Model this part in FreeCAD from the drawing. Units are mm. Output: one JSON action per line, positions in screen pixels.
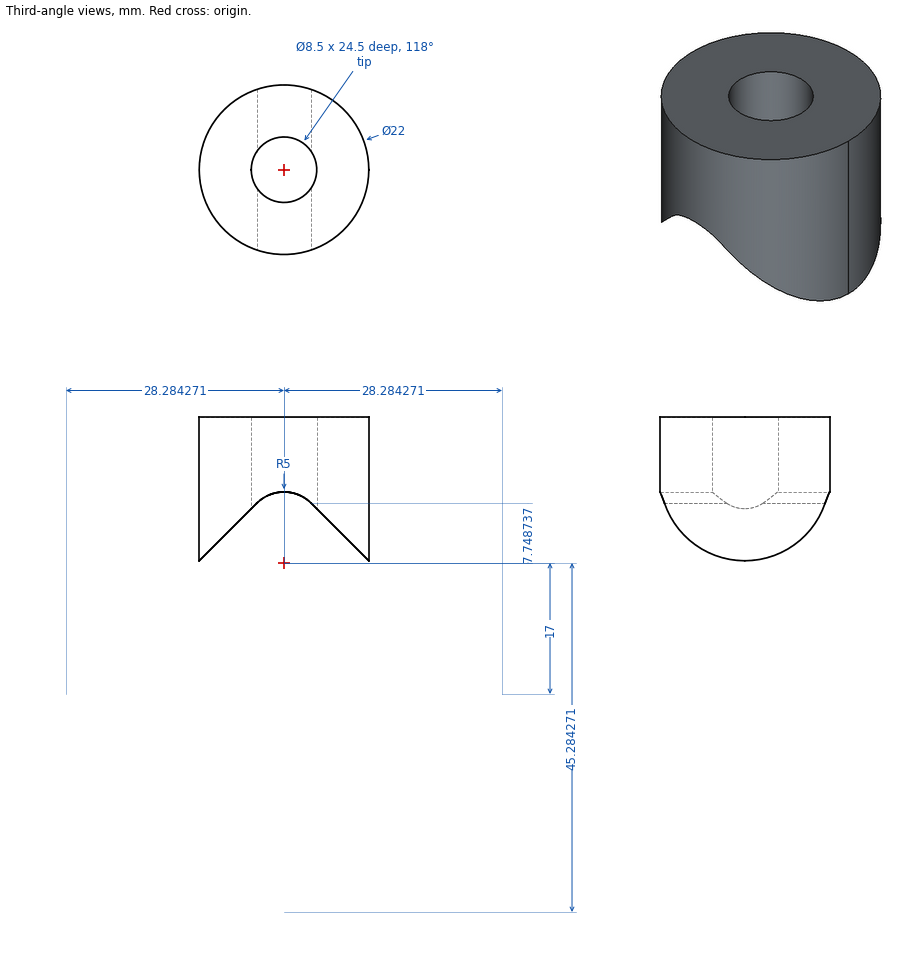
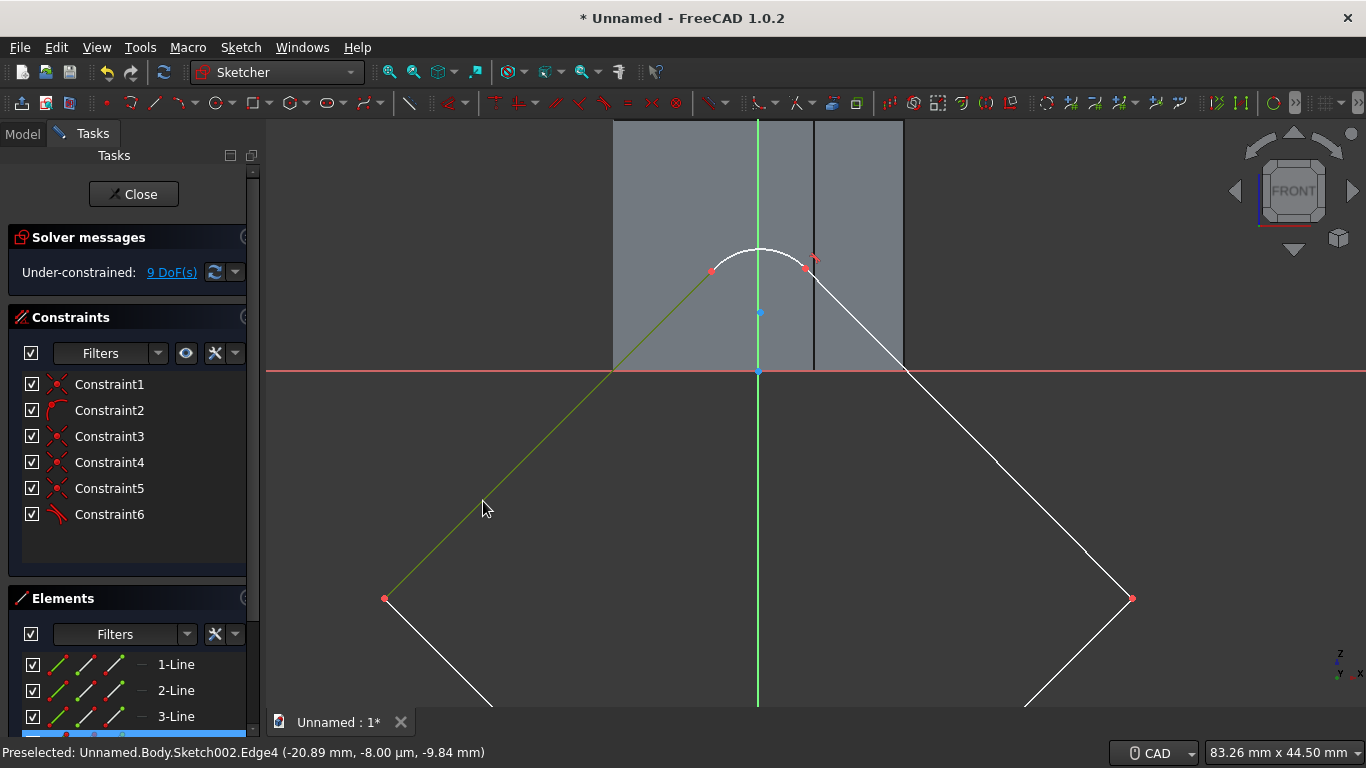
{"action": "left_click", "coordinate": [778, 252]}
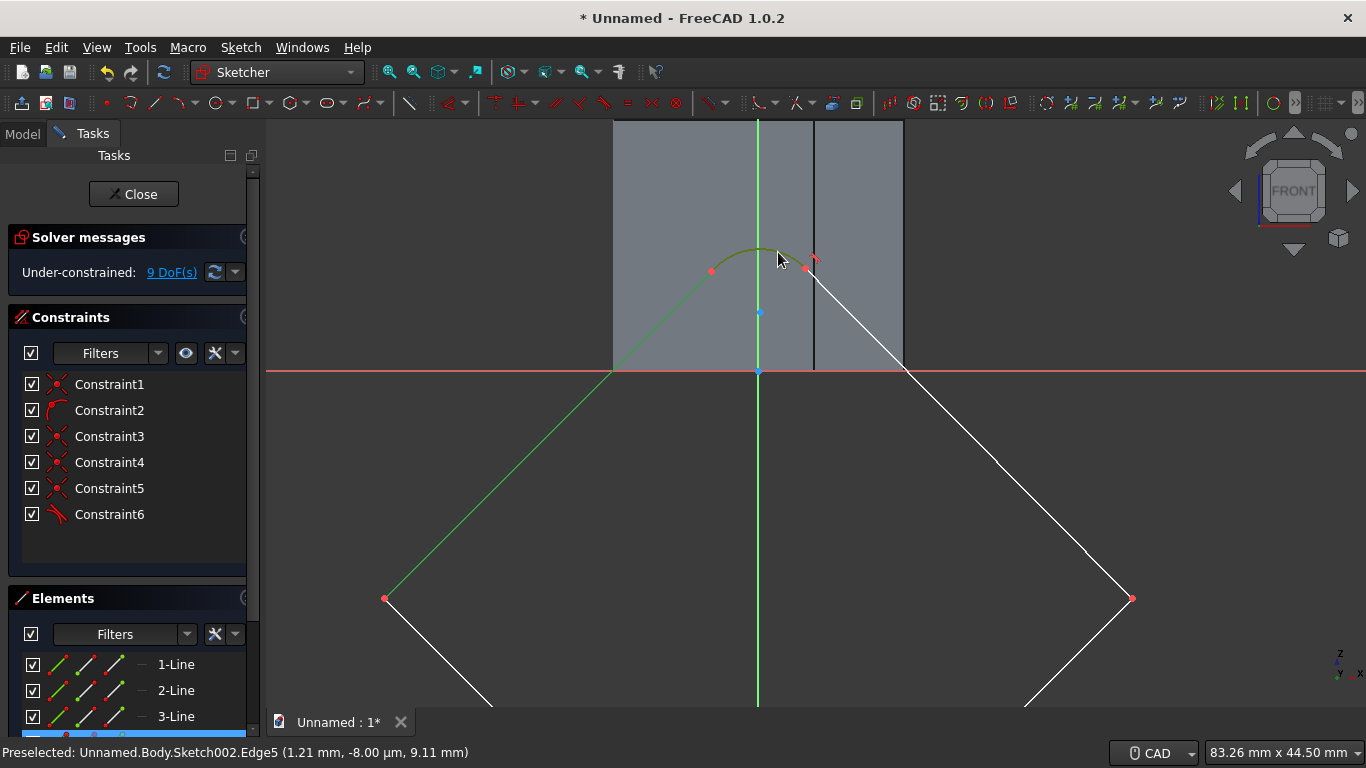
{"action": "left_click", "coordinate": [604, 104]}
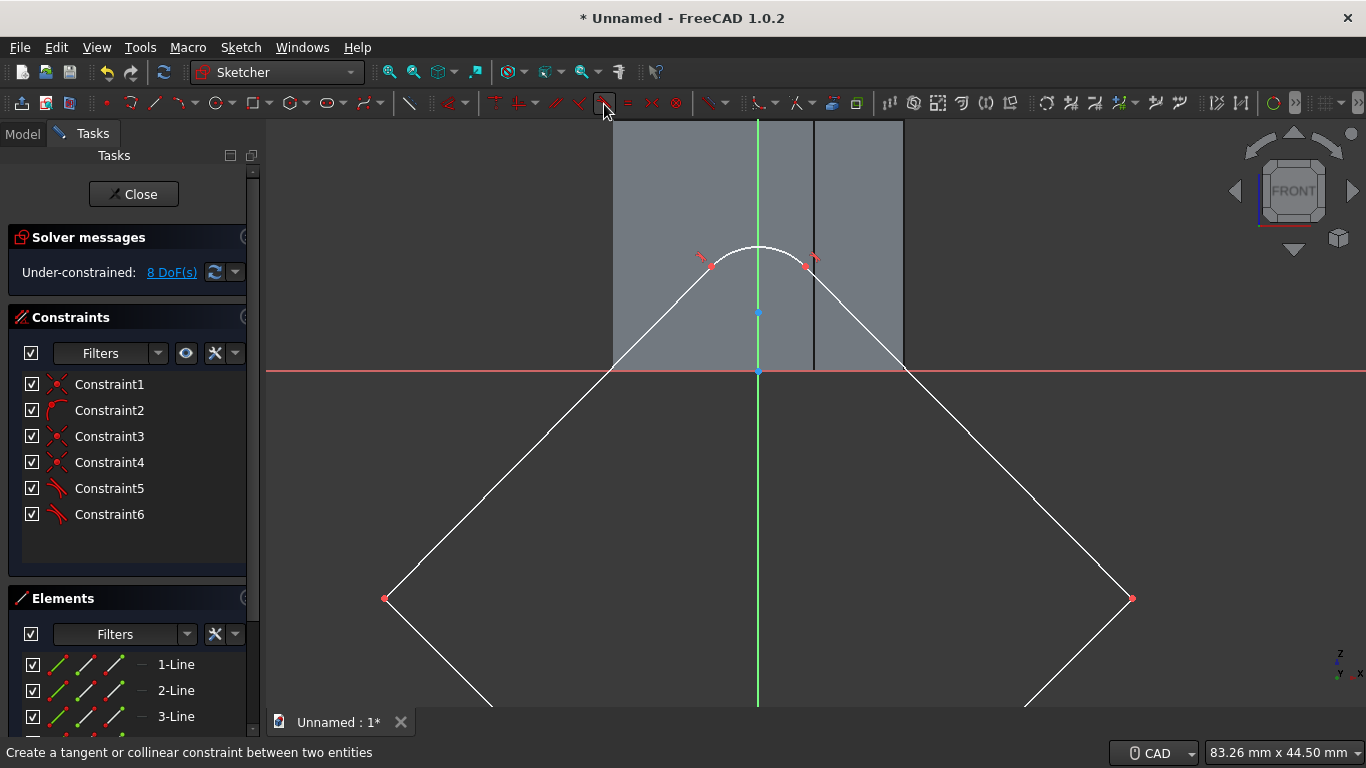
{"action": "left_click", "coordinate": [759, 313]}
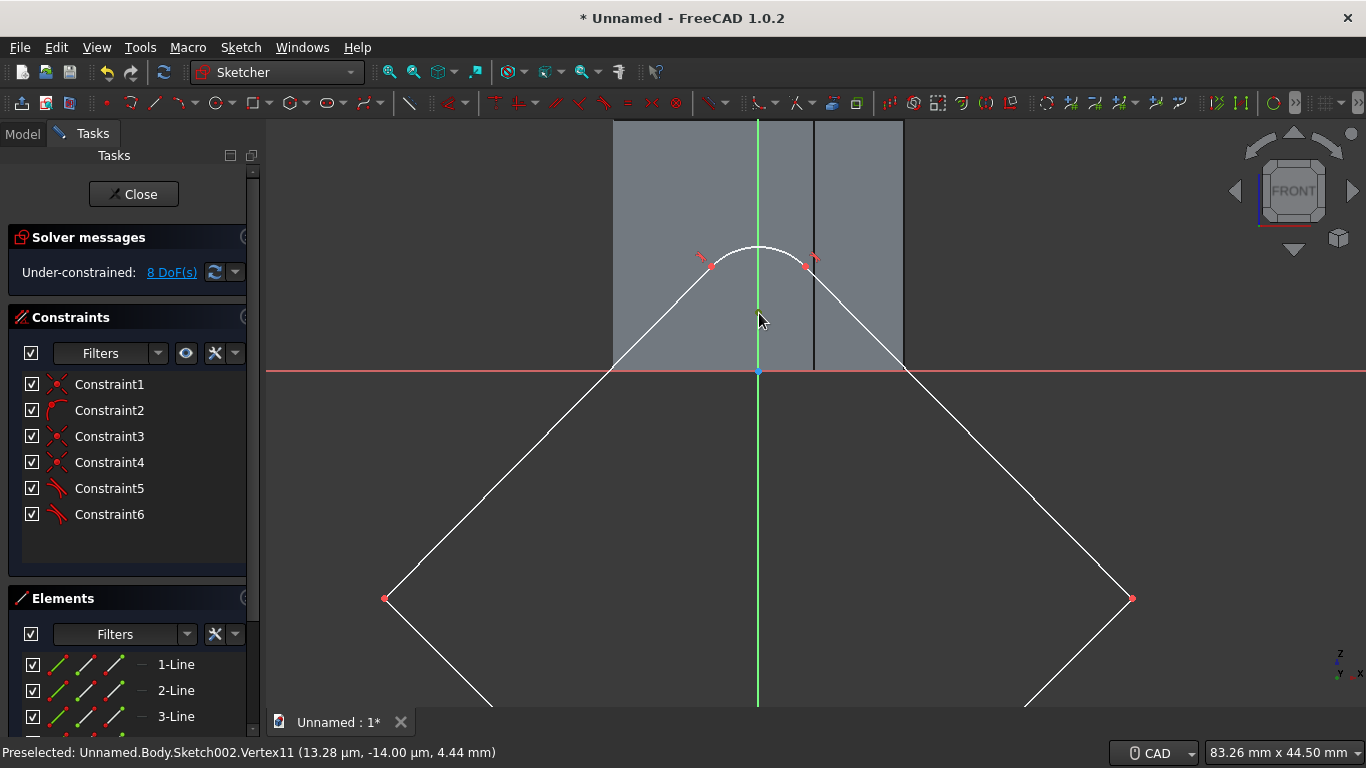
{"action": "left_click", "coordinate": [758, 641]}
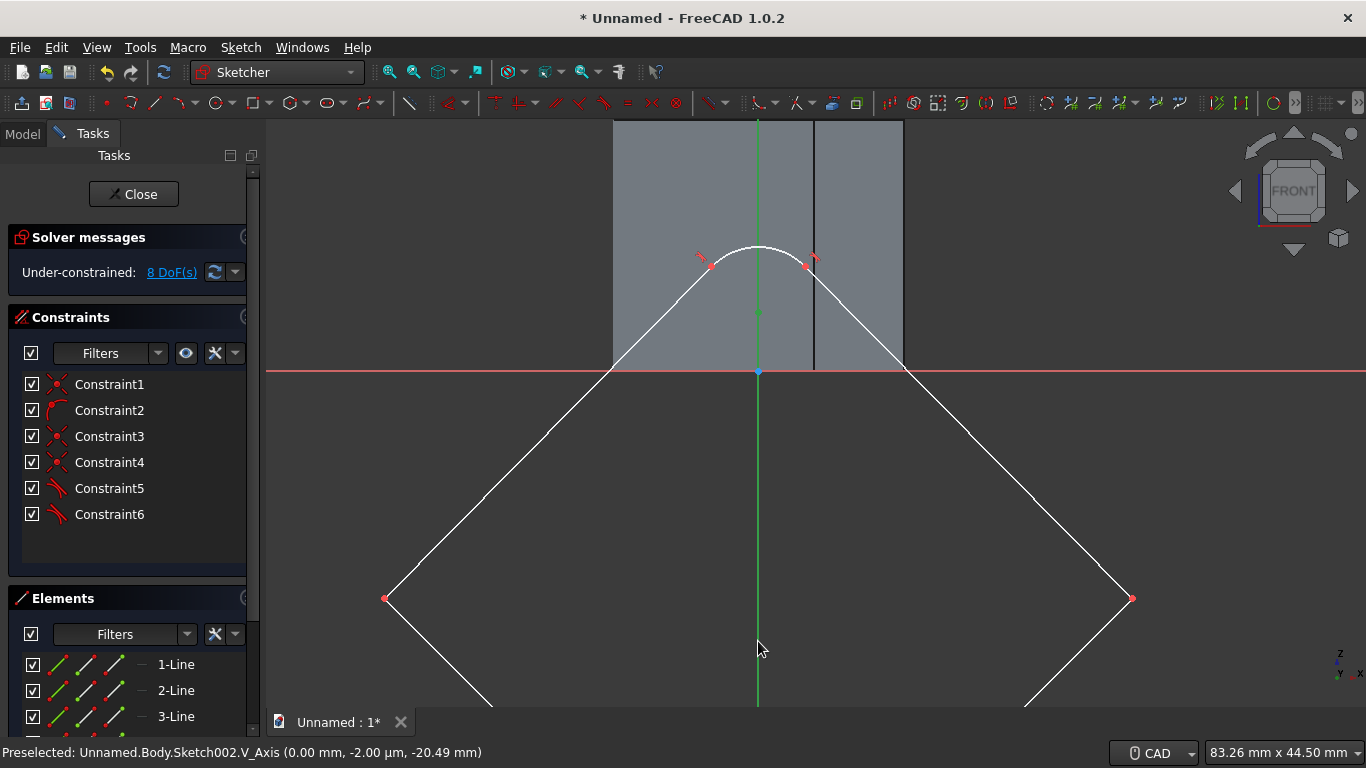
{"action": "key", "text": "c"}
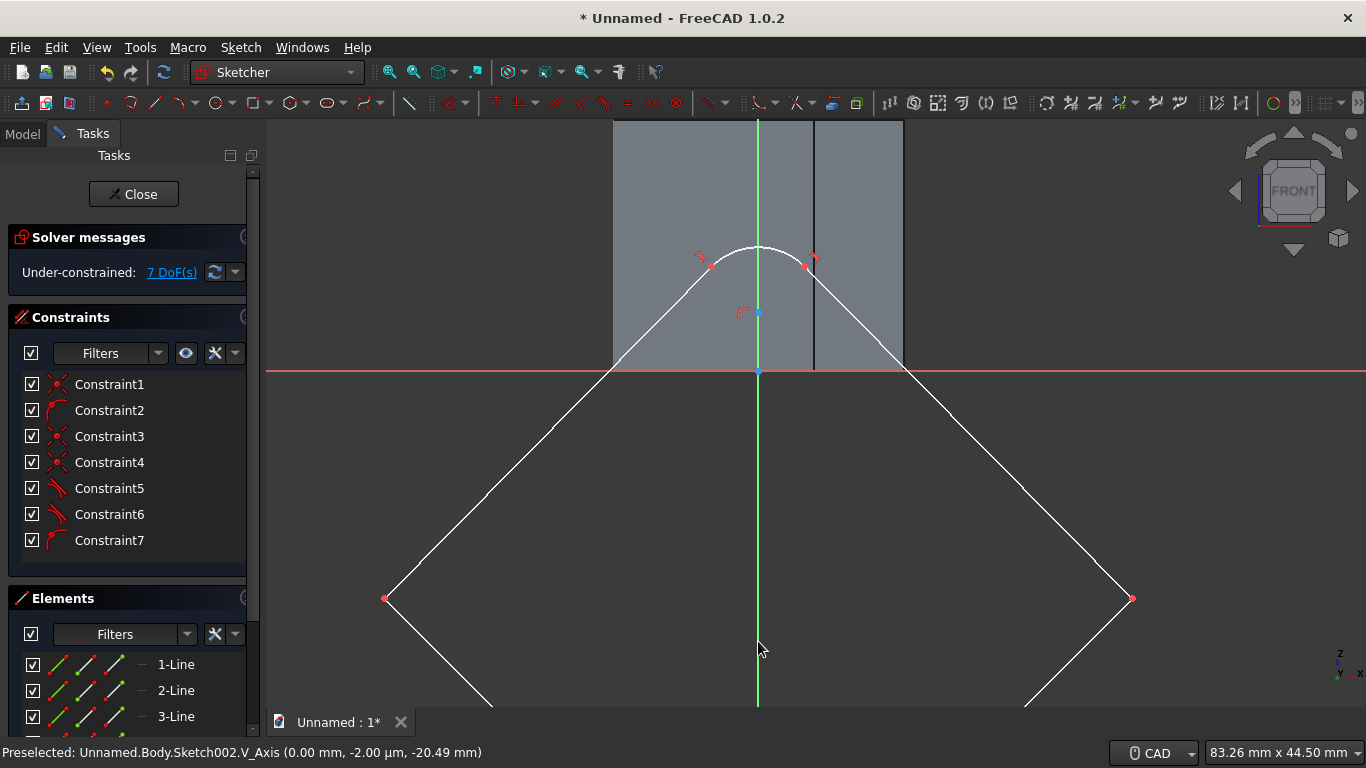
{"action": "left_click", "coordinate": [448, 104]}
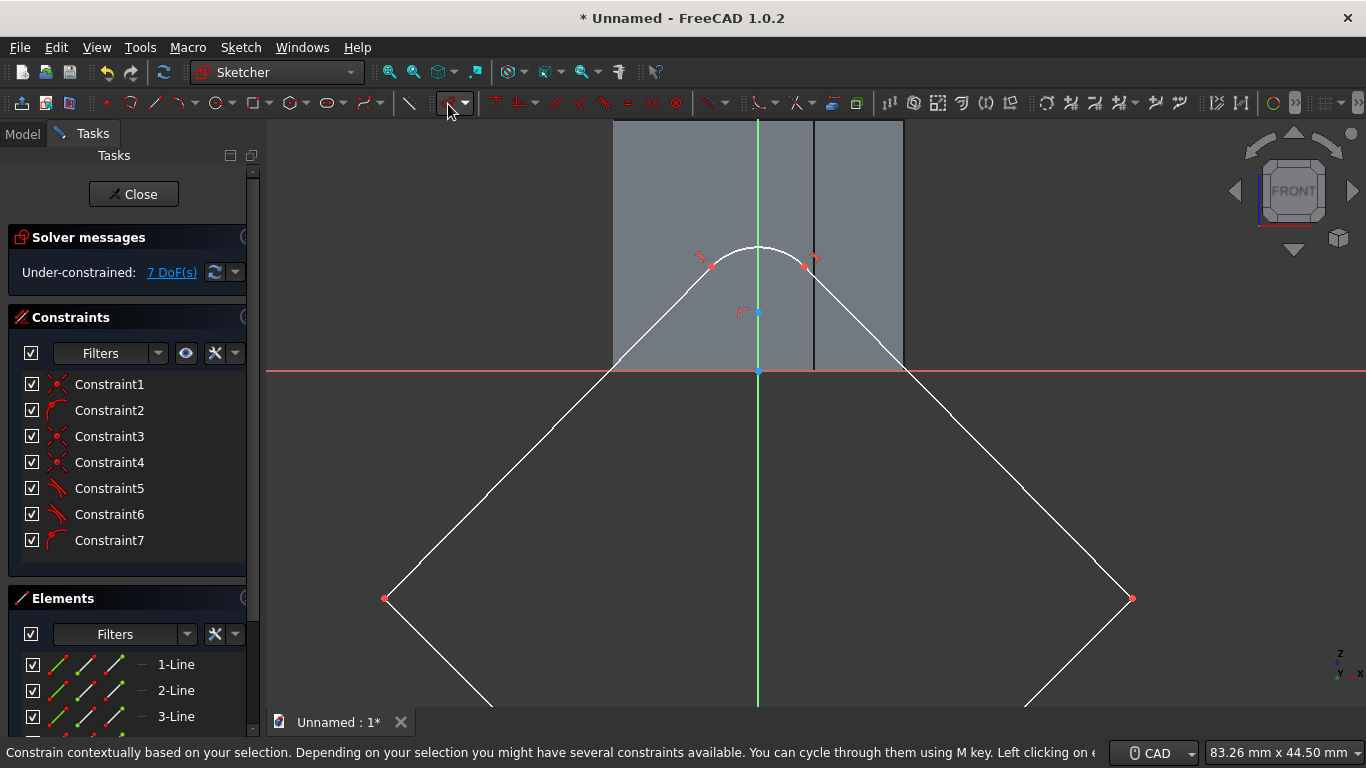
{"action": "left_click", "coordinate": [779, 251]}
{"action": "left_click", "coordinate": [789, 221]}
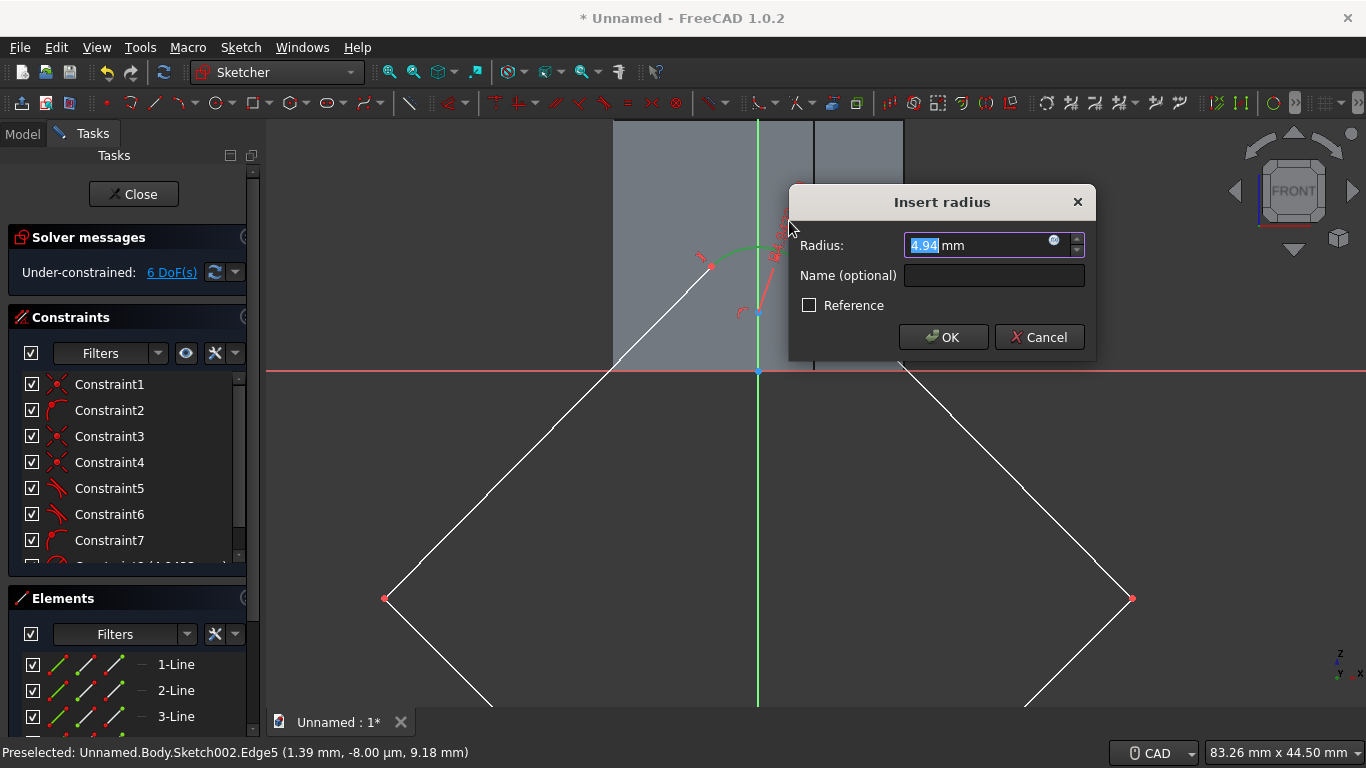
{"action": "type", "text": "5"}
{"action": "key", "text": "Return"}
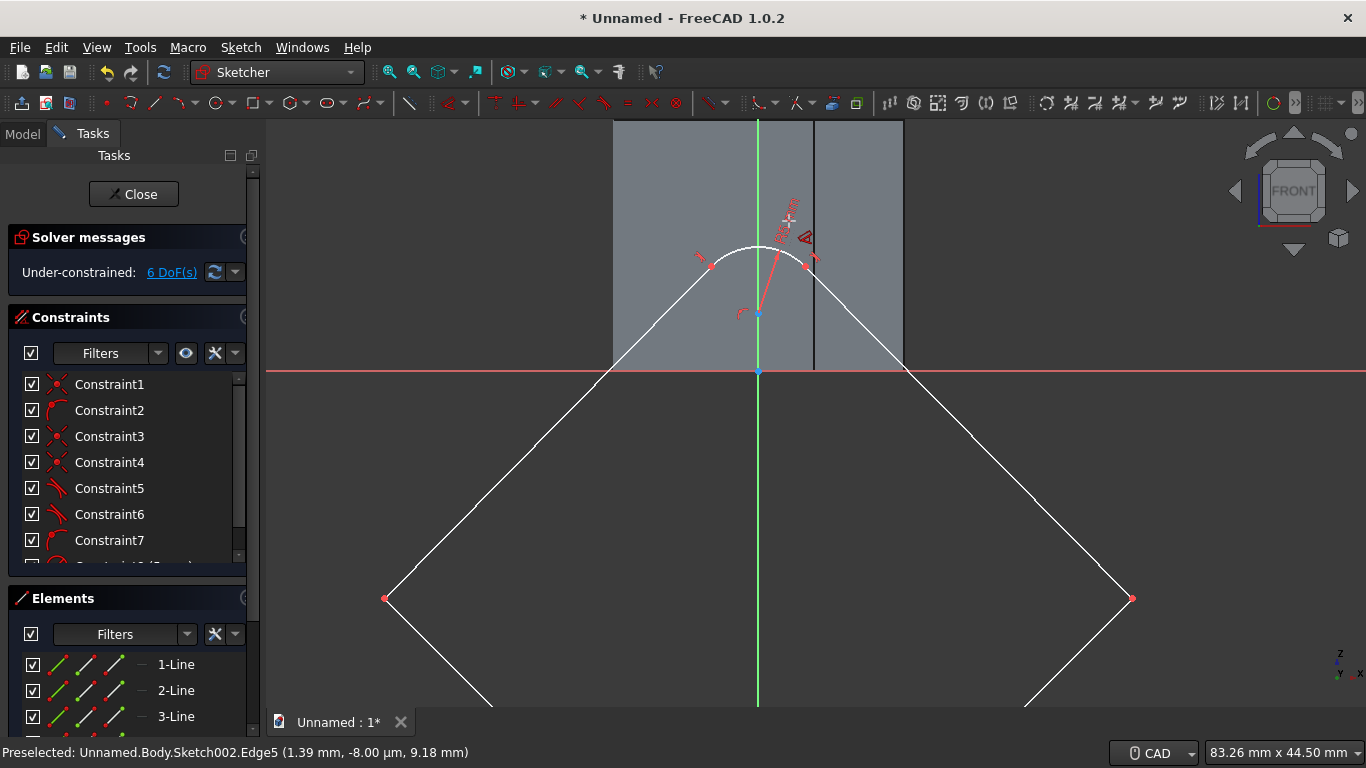
{"action": "left_click", "coordinate": [1132, 599]}
{"action": "left_click", "coordinate": [1166, 485]}